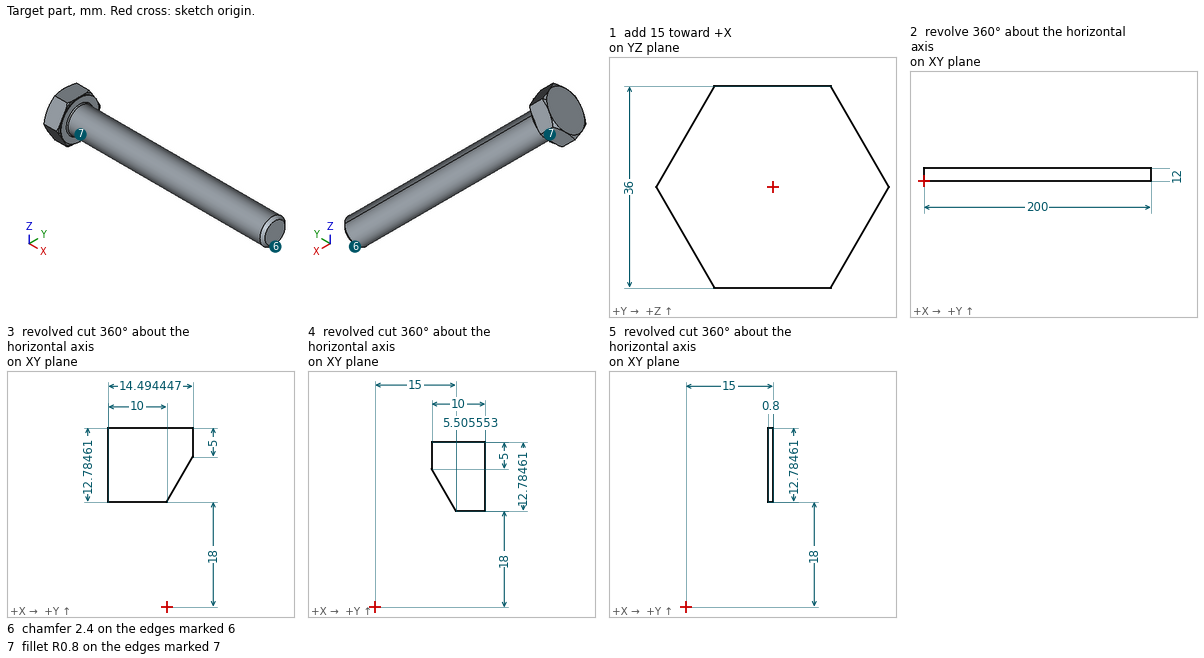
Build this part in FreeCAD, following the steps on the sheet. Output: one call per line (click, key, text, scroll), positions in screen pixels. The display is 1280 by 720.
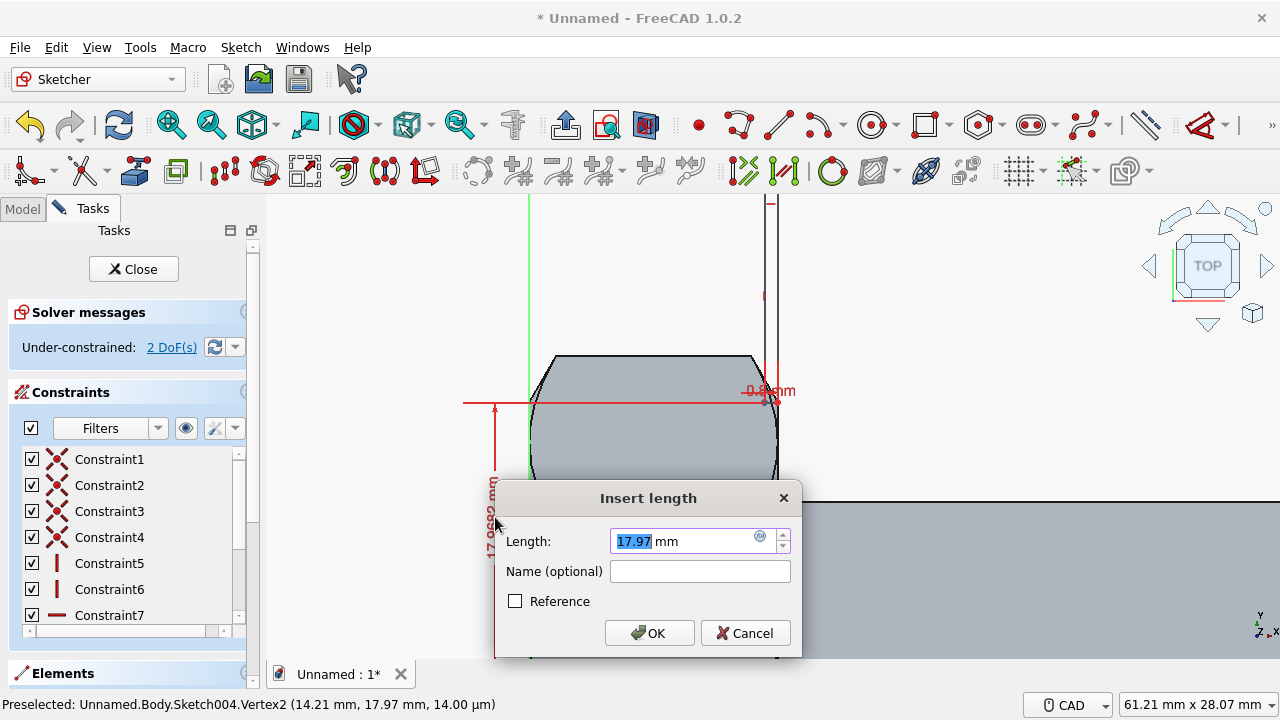
text(18)
key(Return)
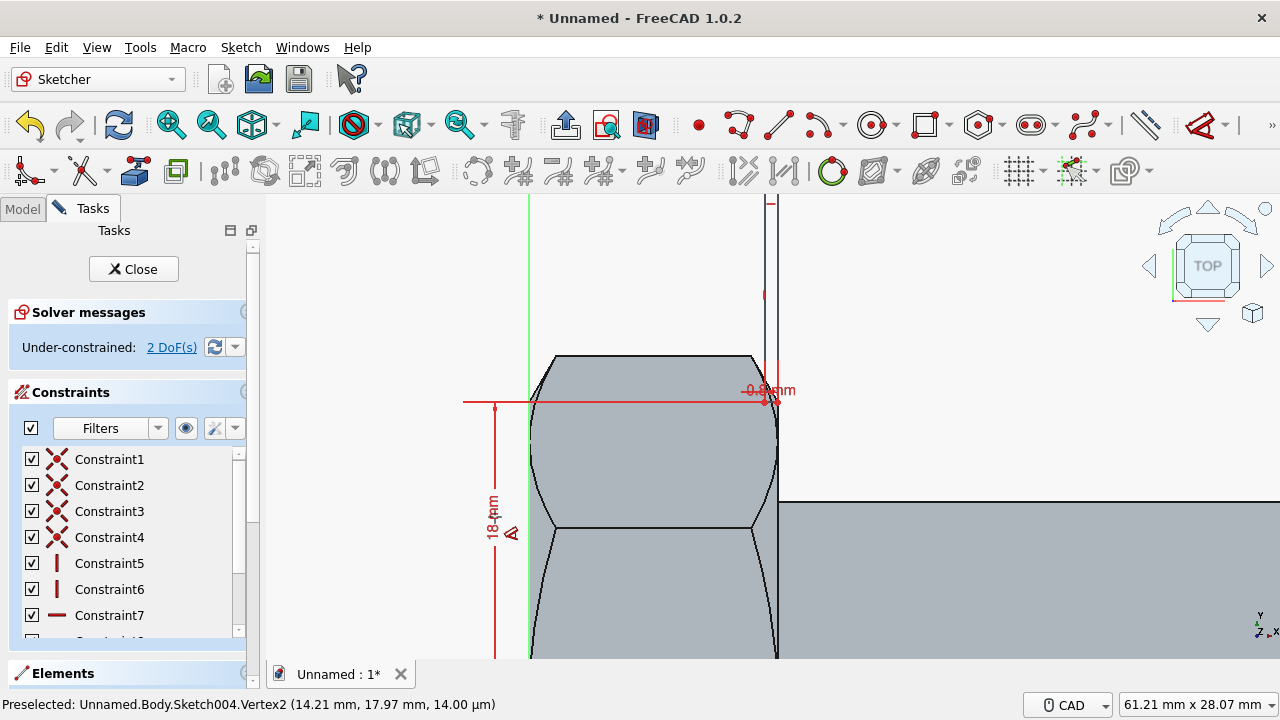
click(778, 402)
click(654, 368)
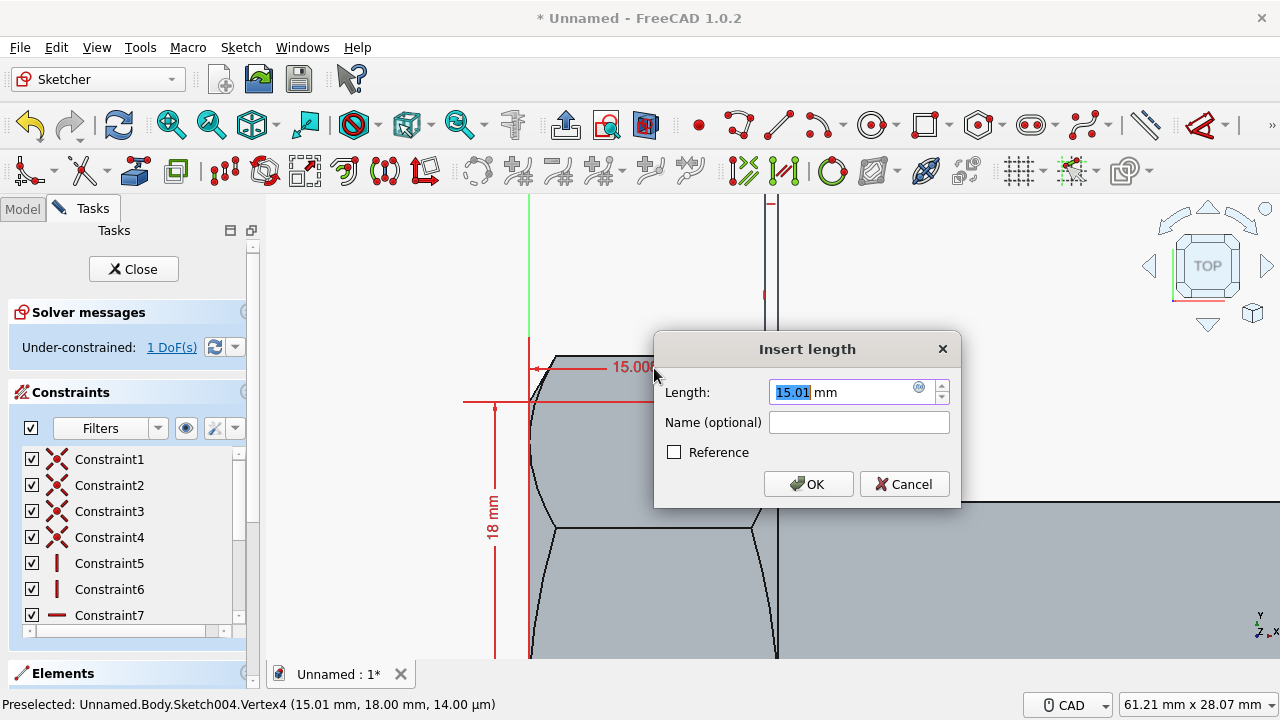
text(15)
key(Return)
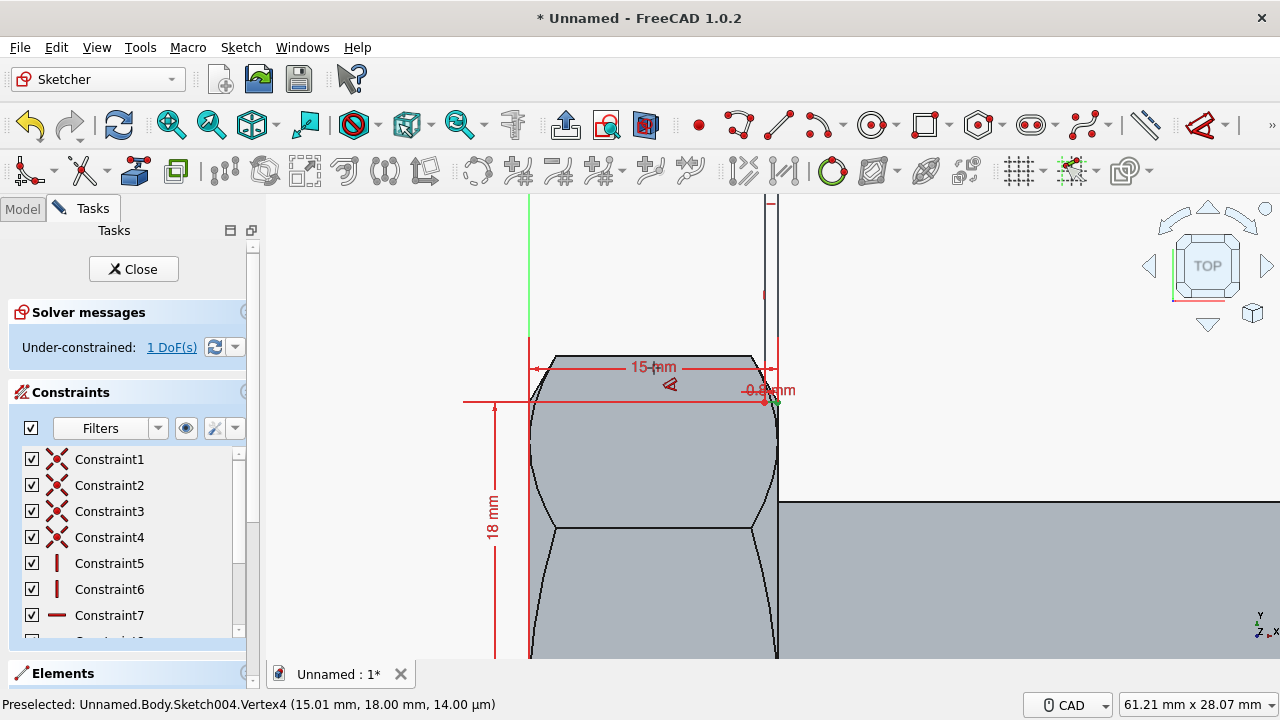
click(765, 255)
click(799, 312)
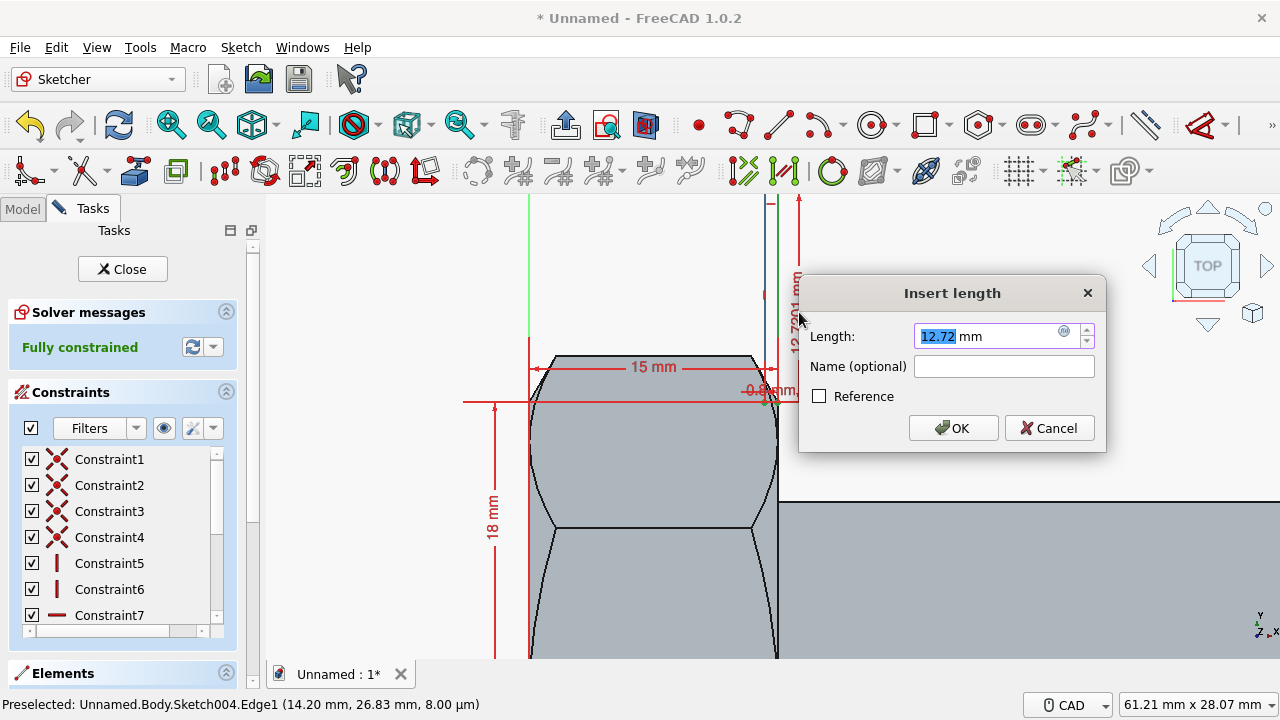
text(12.78461)
key(Return)
key(Escape)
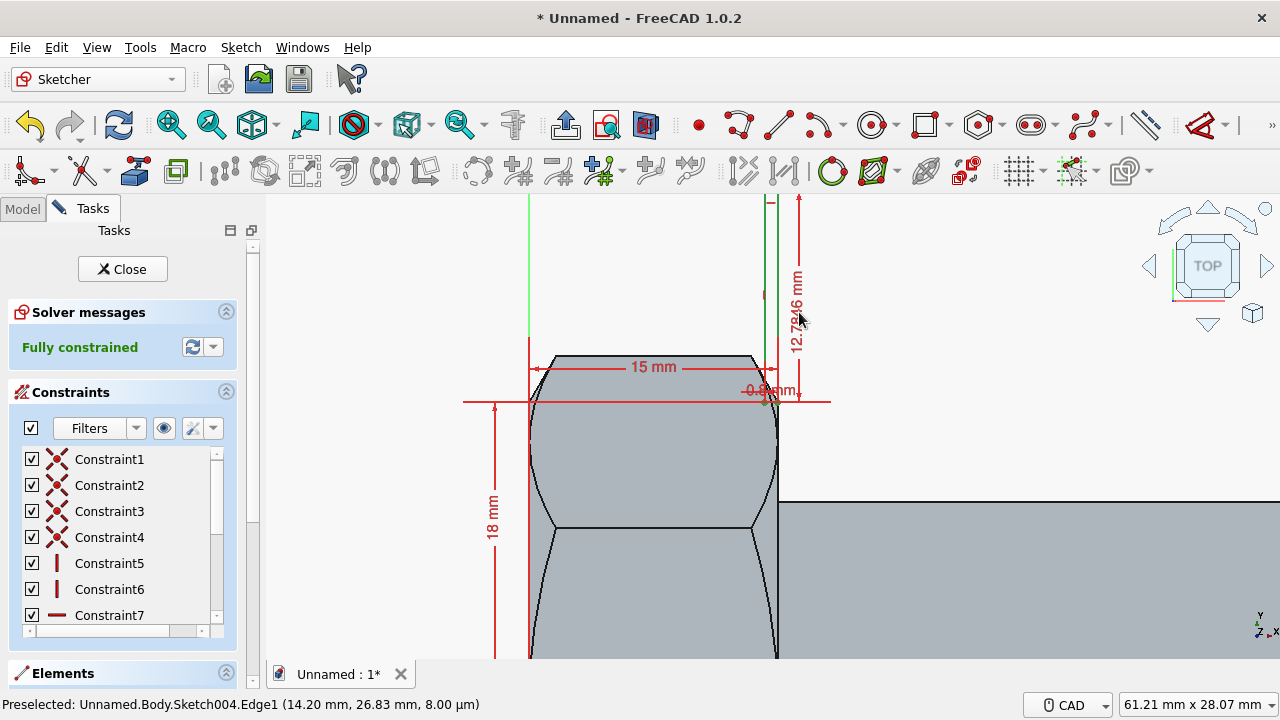
click(123, 269)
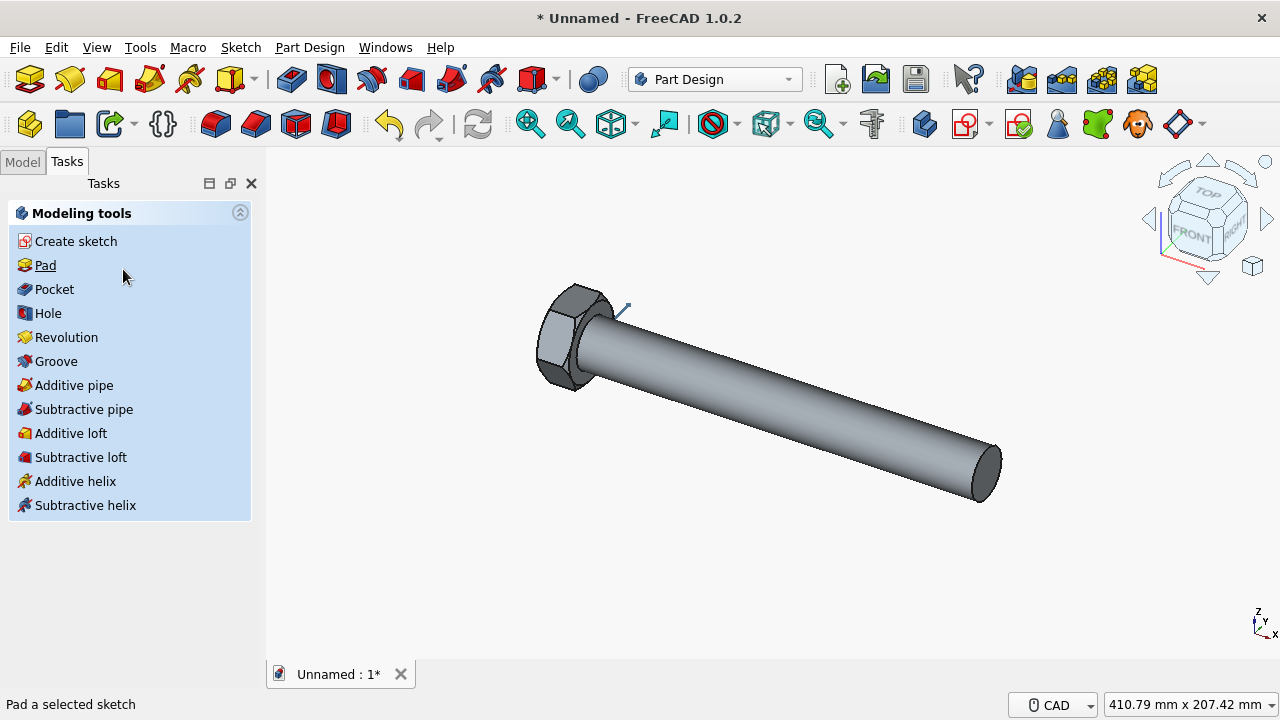
click(372, 80)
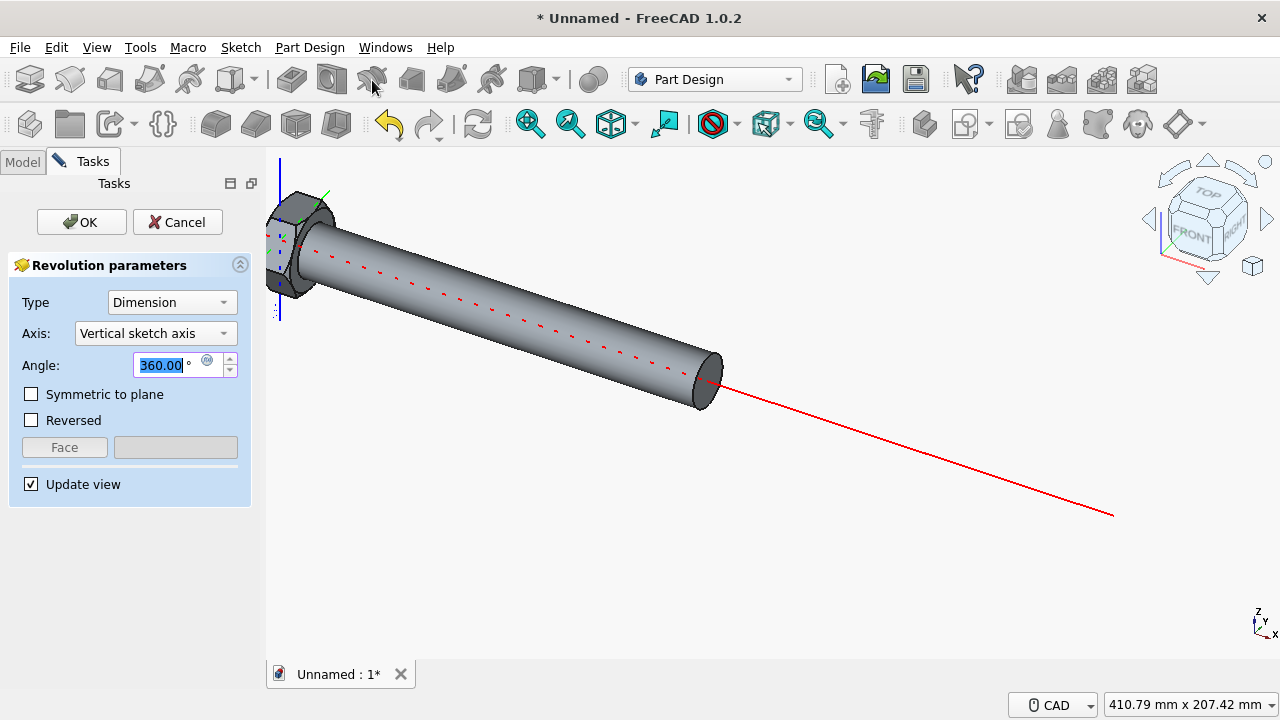
click(156, 334)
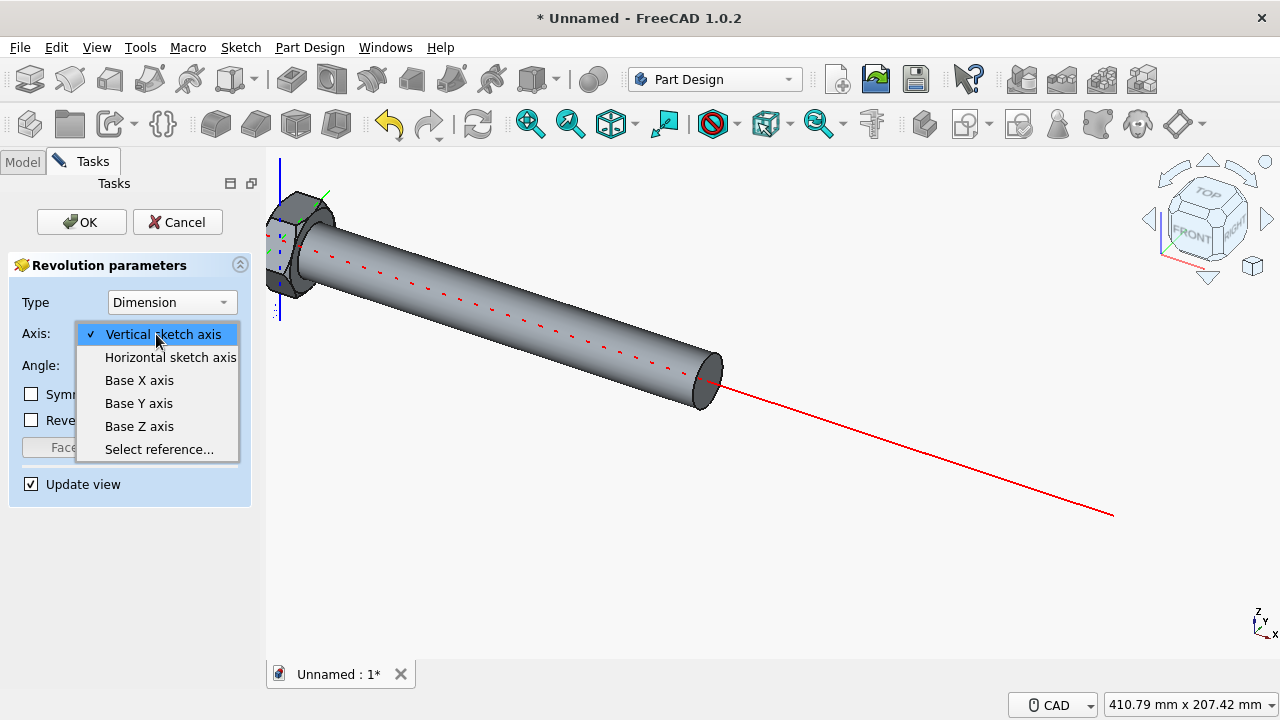
click(156, 358)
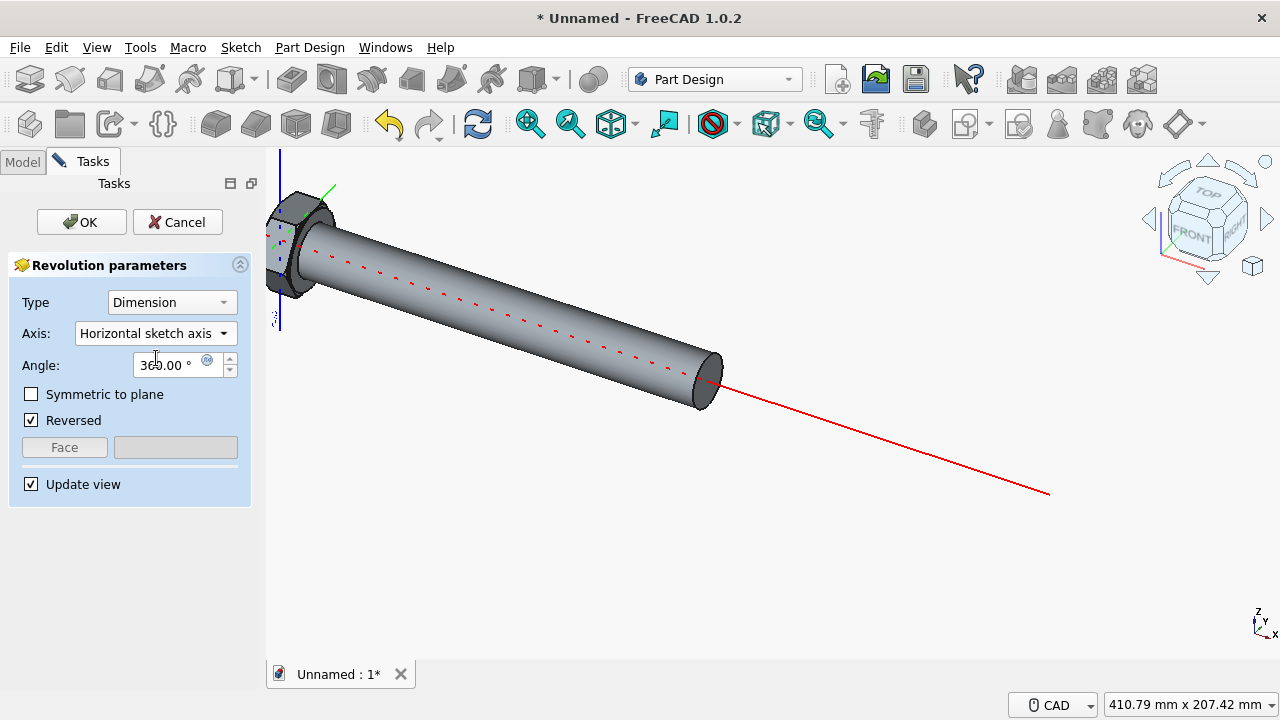
click(82, 222)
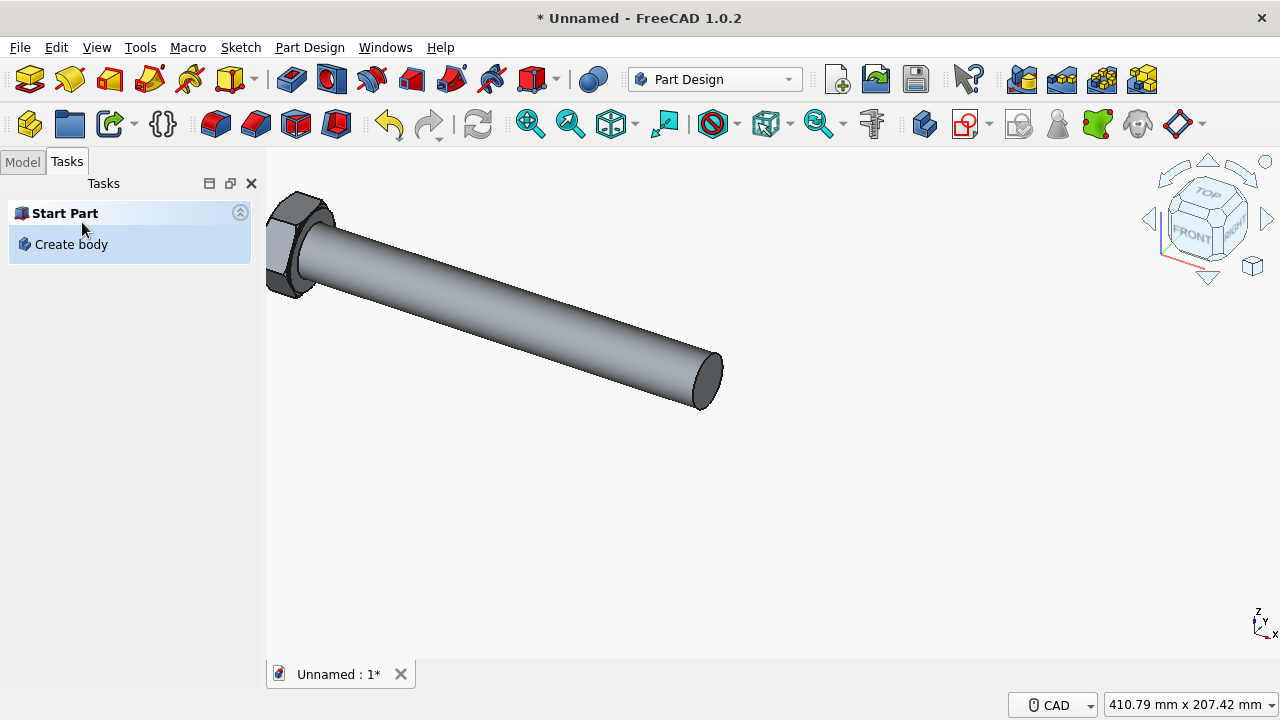
key(v)
key(f)